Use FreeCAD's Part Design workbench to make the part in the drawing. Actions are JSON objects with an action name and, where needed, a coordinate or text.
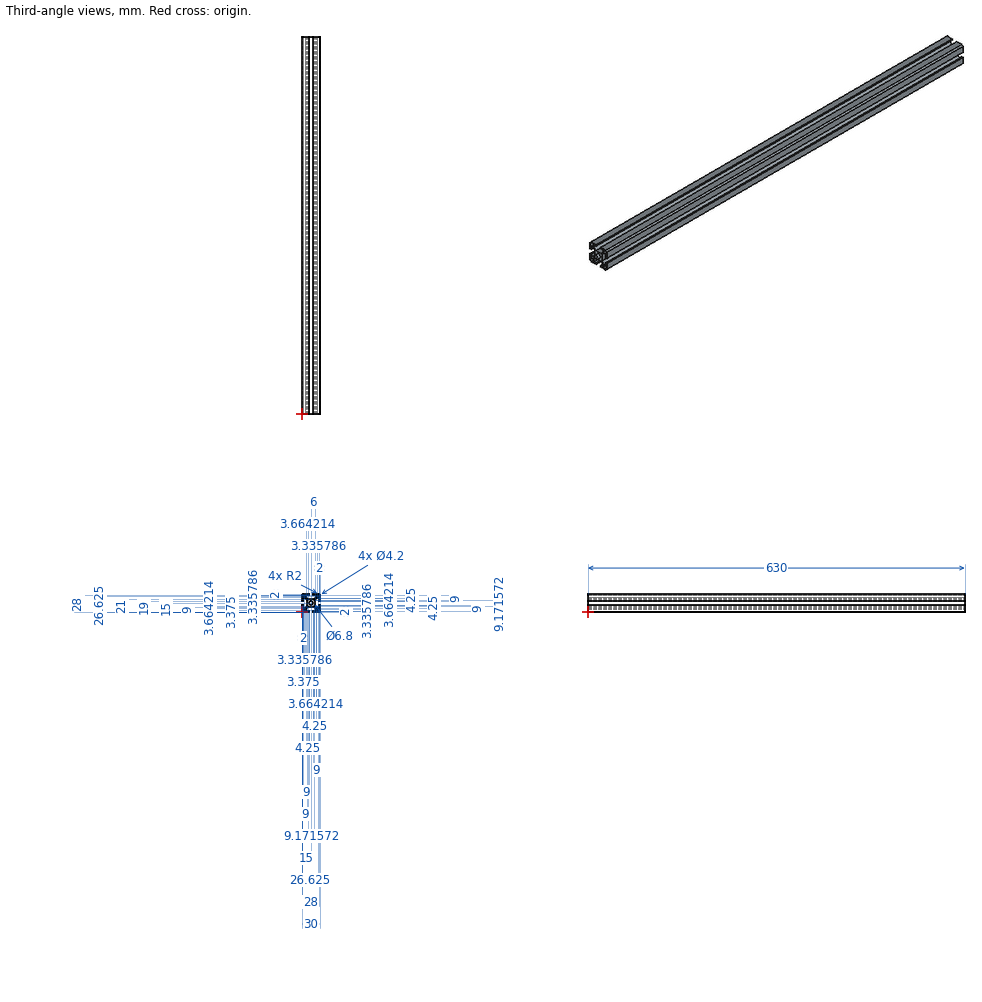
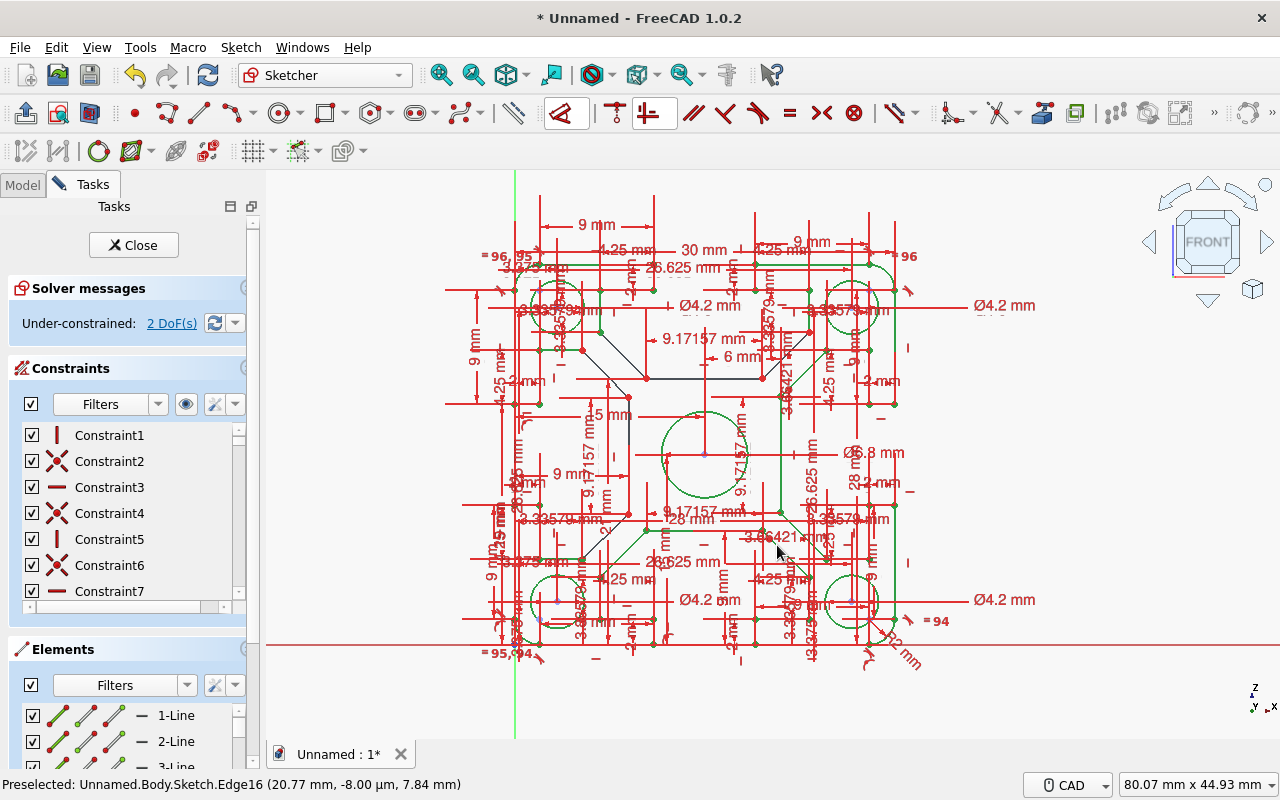
{"action": "left_click", "coordinate": [596, 546]}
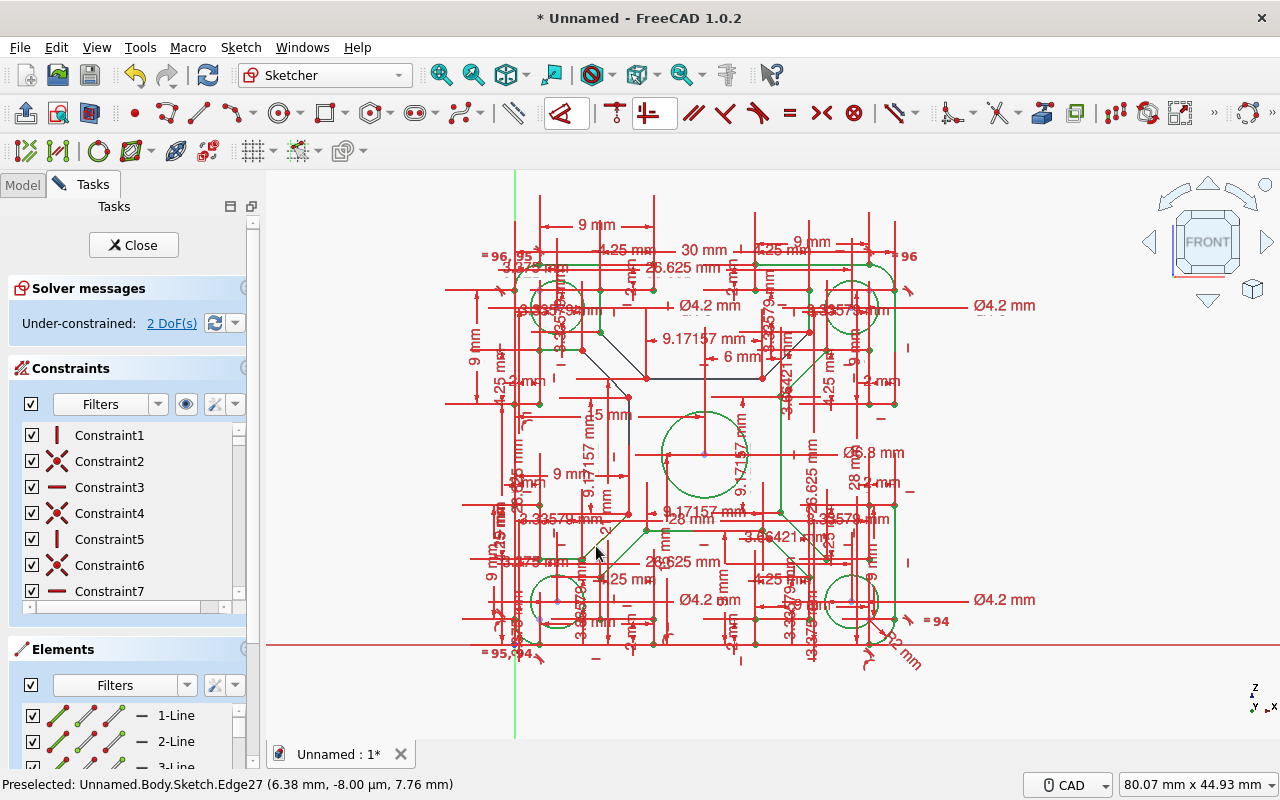
{"action": "key", "text": "i"}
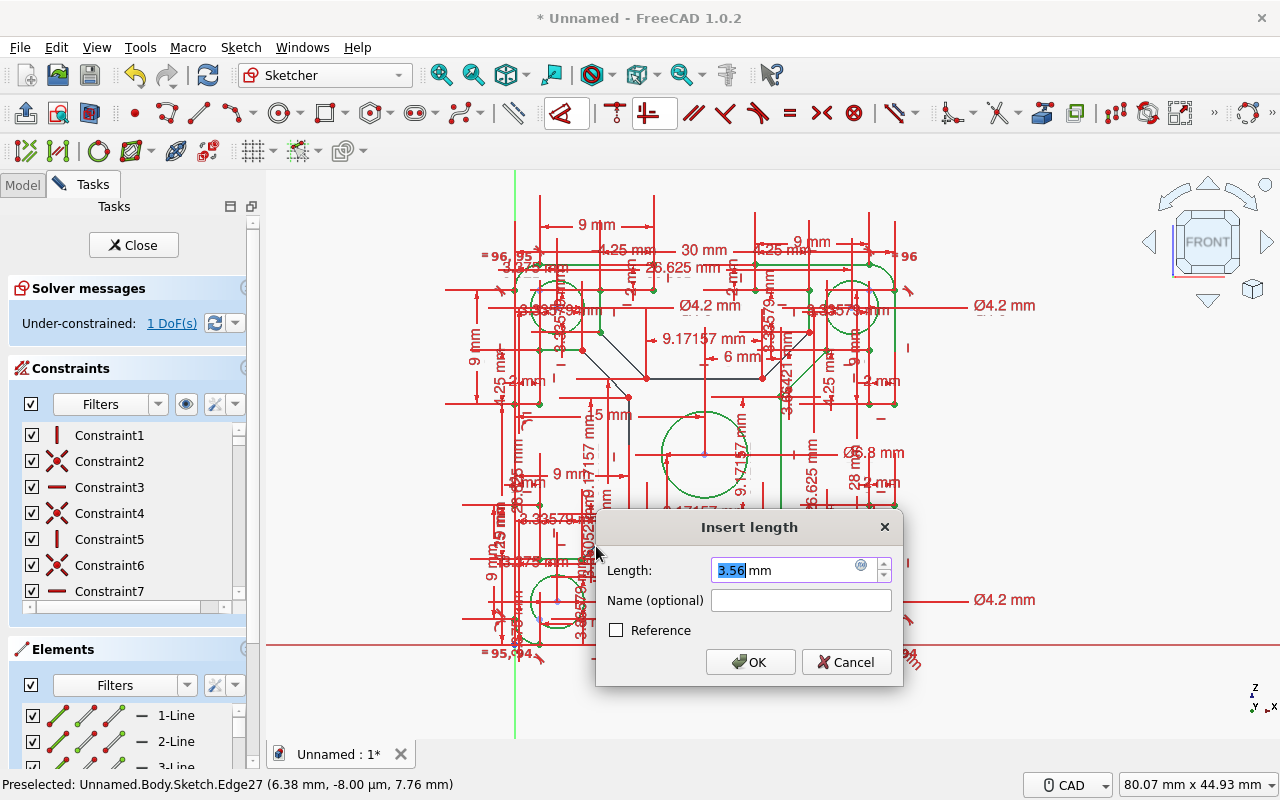
{"action": "type", "text": "3.664214"}
{"action": "key", "text": "Return"}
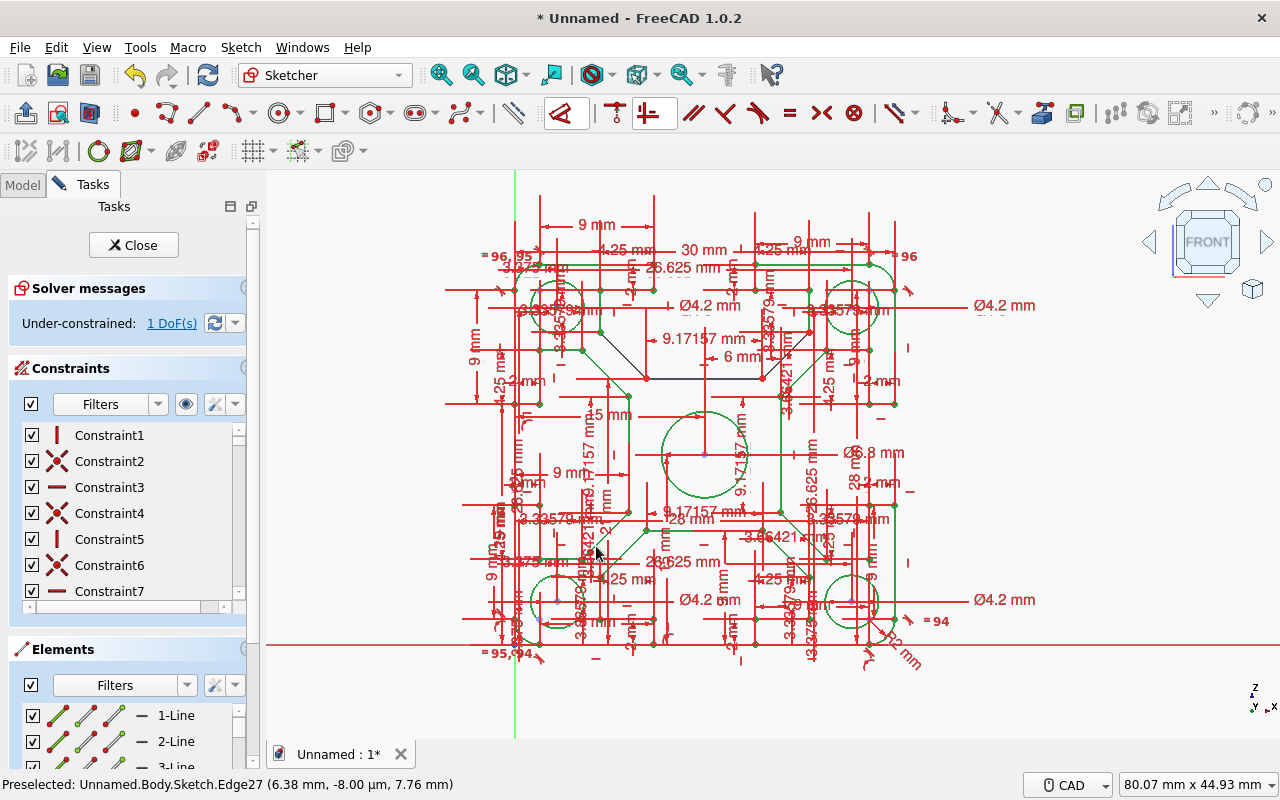
{"action": "left_click", "coordinate": [614, 346]}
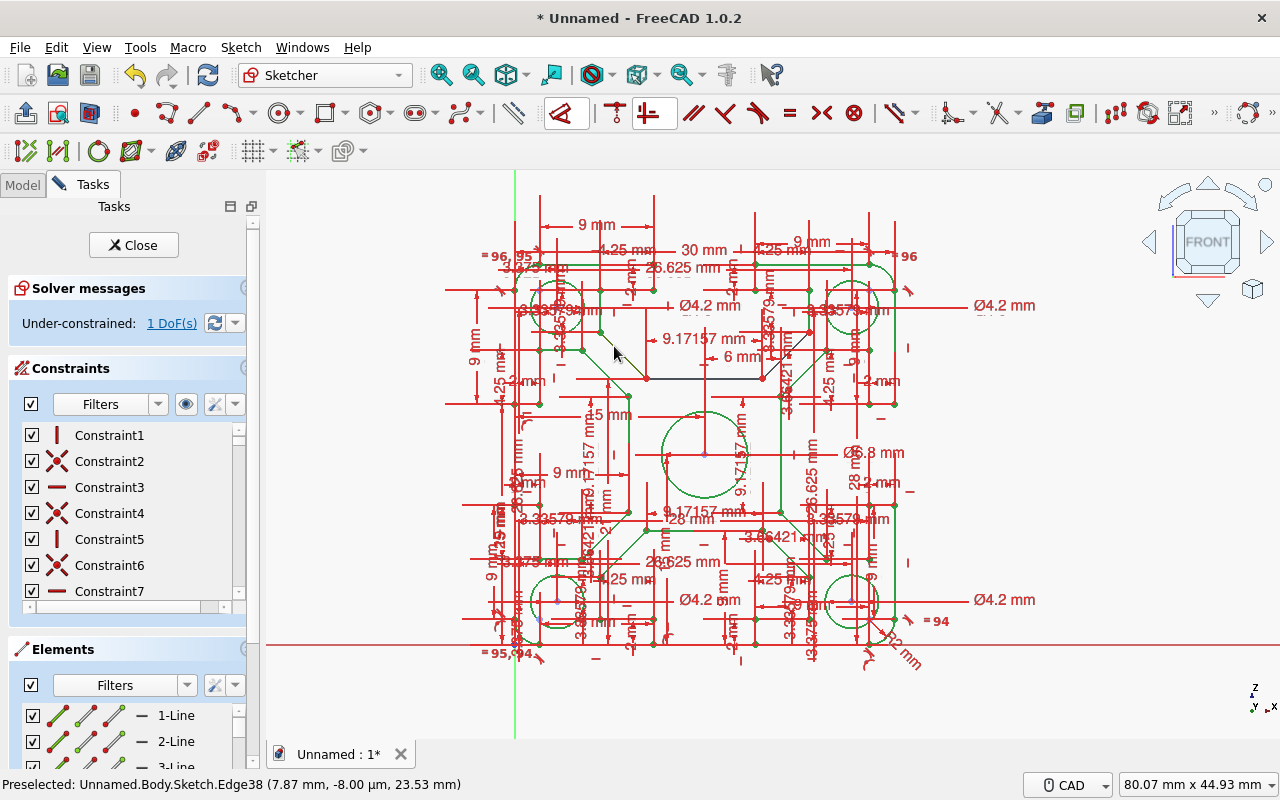
{"action": "left_click", "coordinate": [584, 114]}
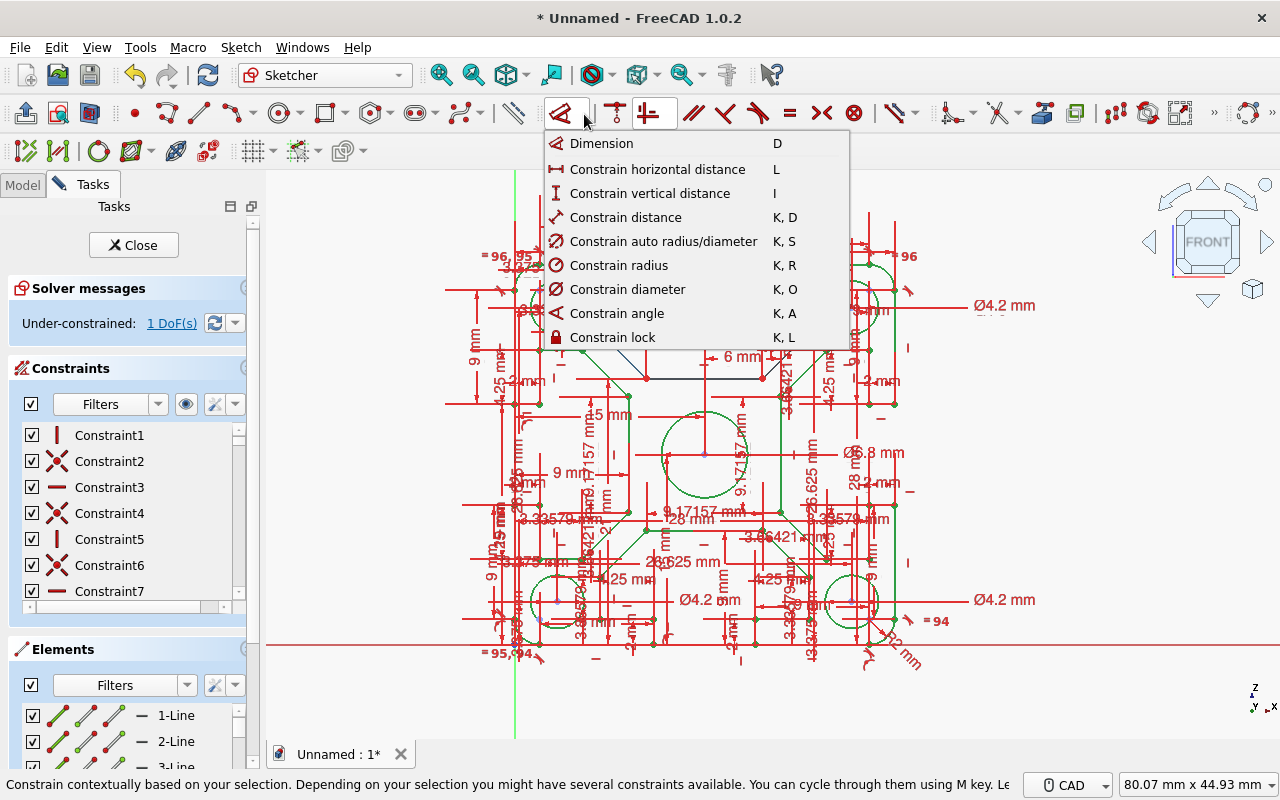
{"action": "left_click", "coordinate": [697, 169]}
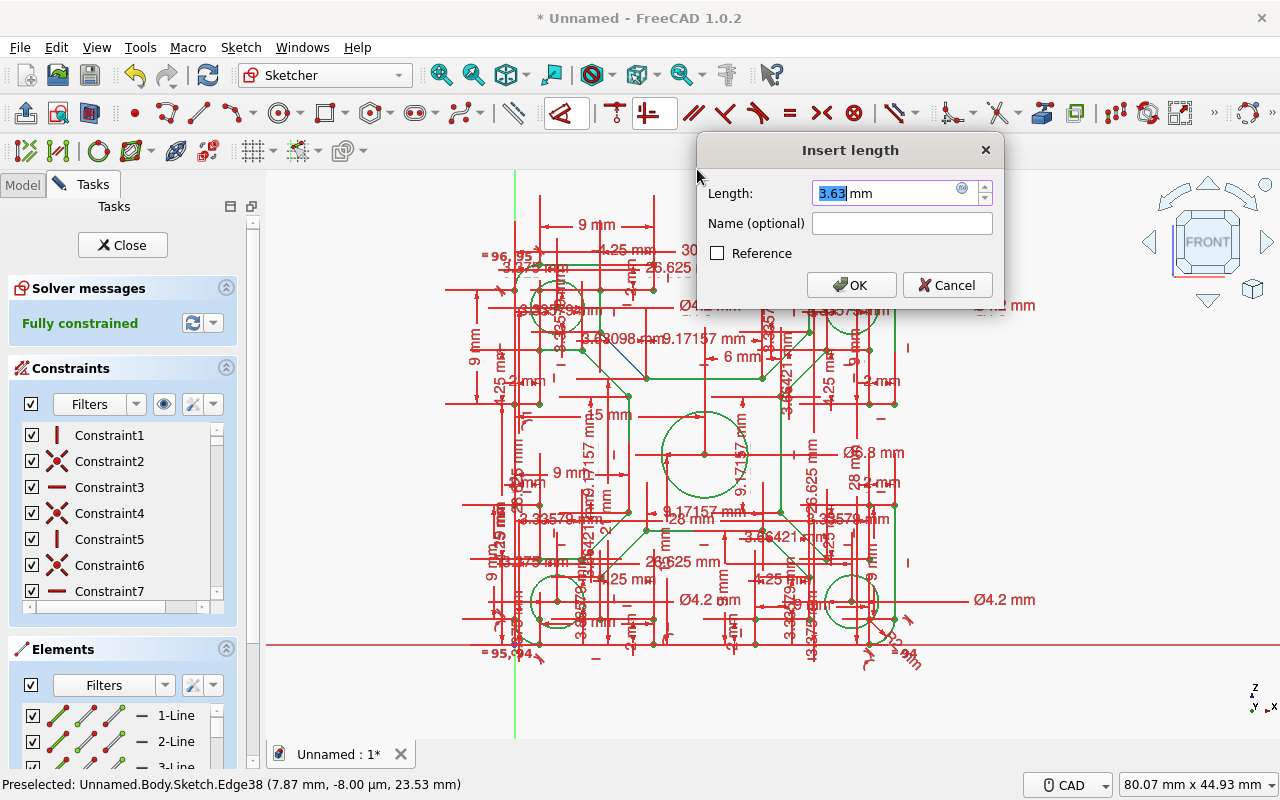
{"action": "type", "text": "3.664214"}
{"action": "key", "text": "Return"}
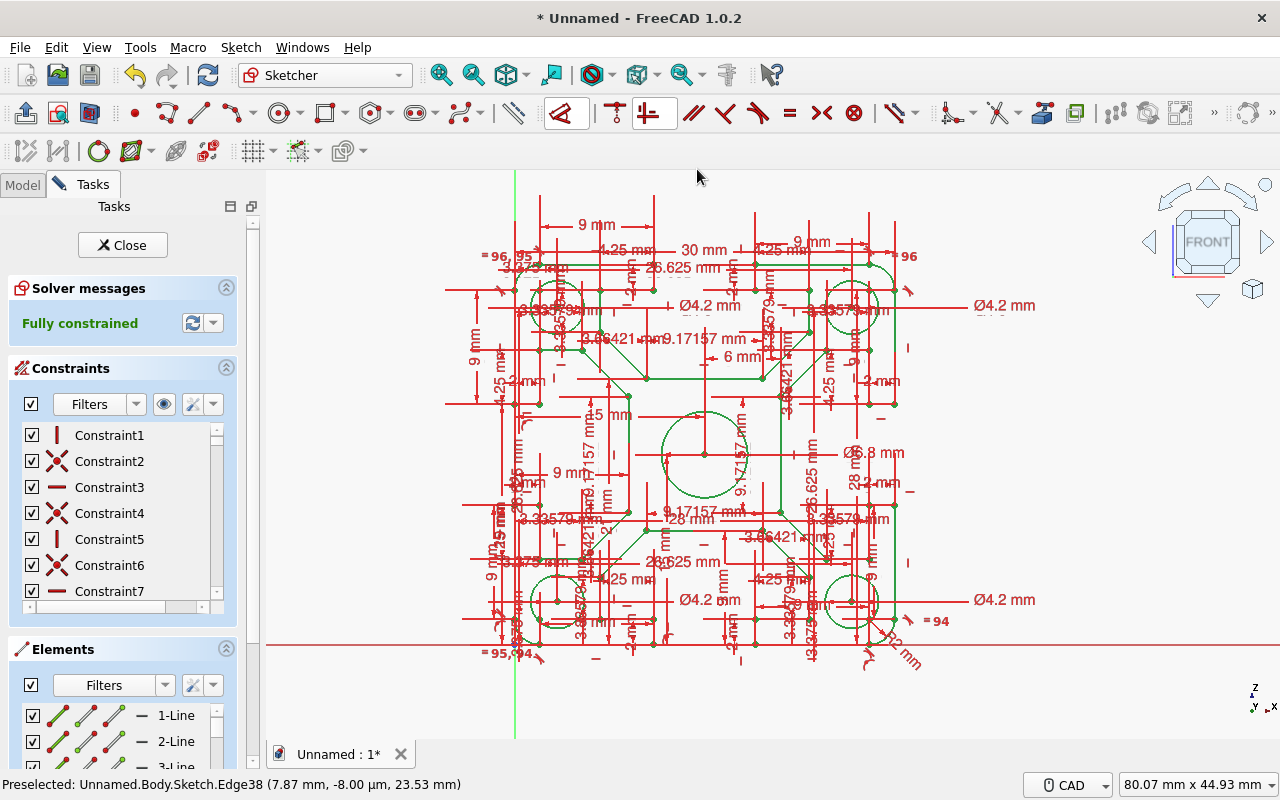
{"action": "left_click", "coordinate": [123, 245]}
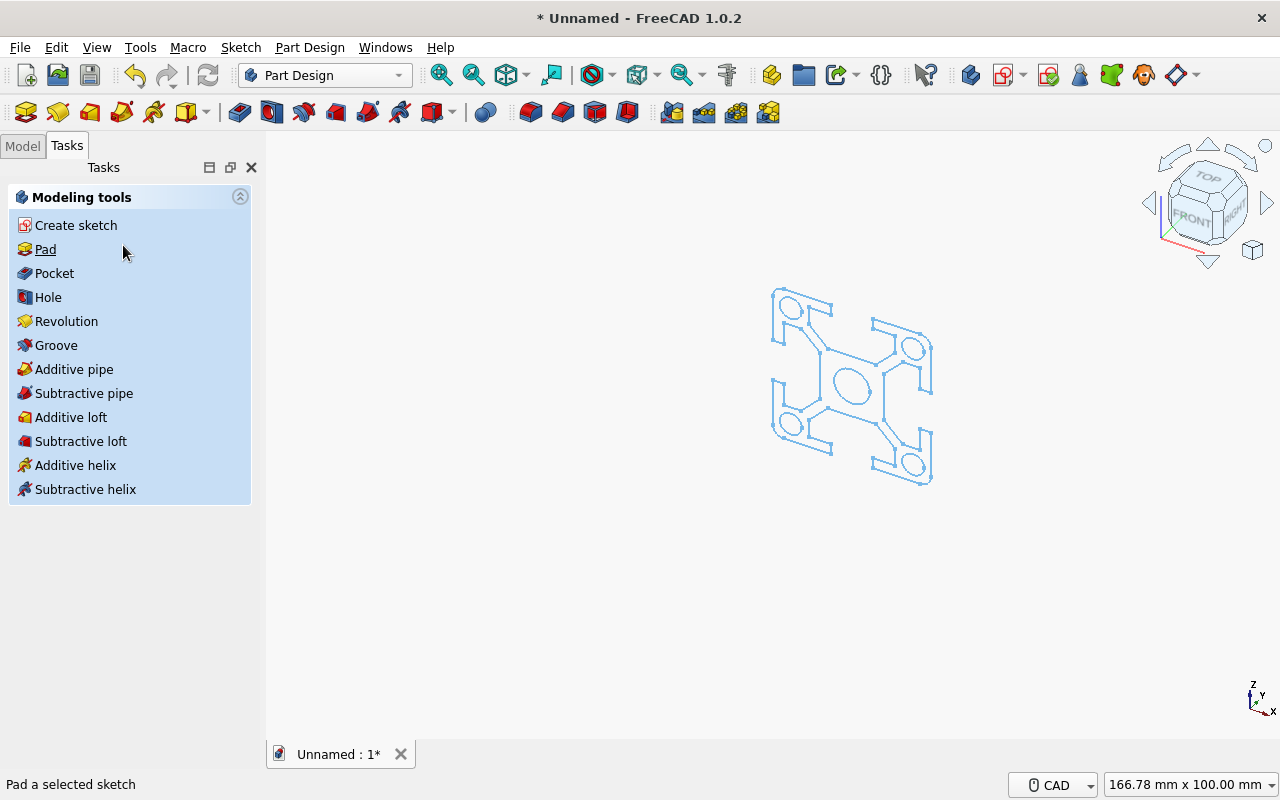
{"action": "left_click", "coordinate": [26, 112]}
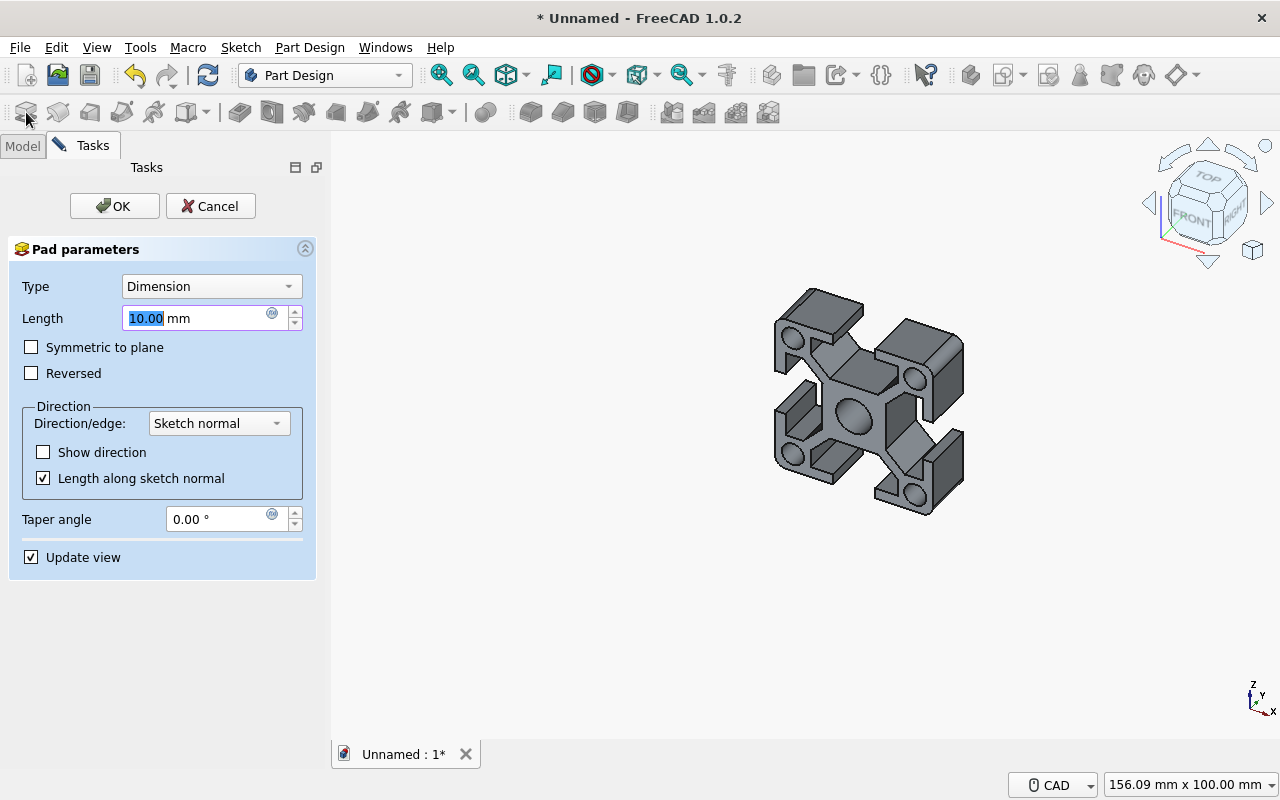
{"action": "type", "text": "630"}
{"action": "key", "text": "Tab"}